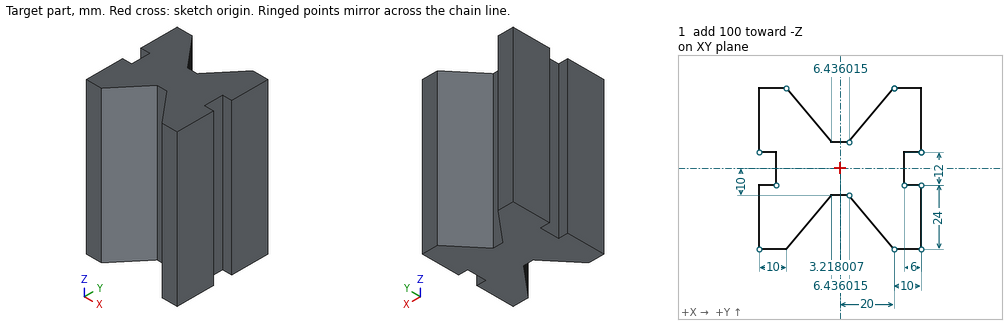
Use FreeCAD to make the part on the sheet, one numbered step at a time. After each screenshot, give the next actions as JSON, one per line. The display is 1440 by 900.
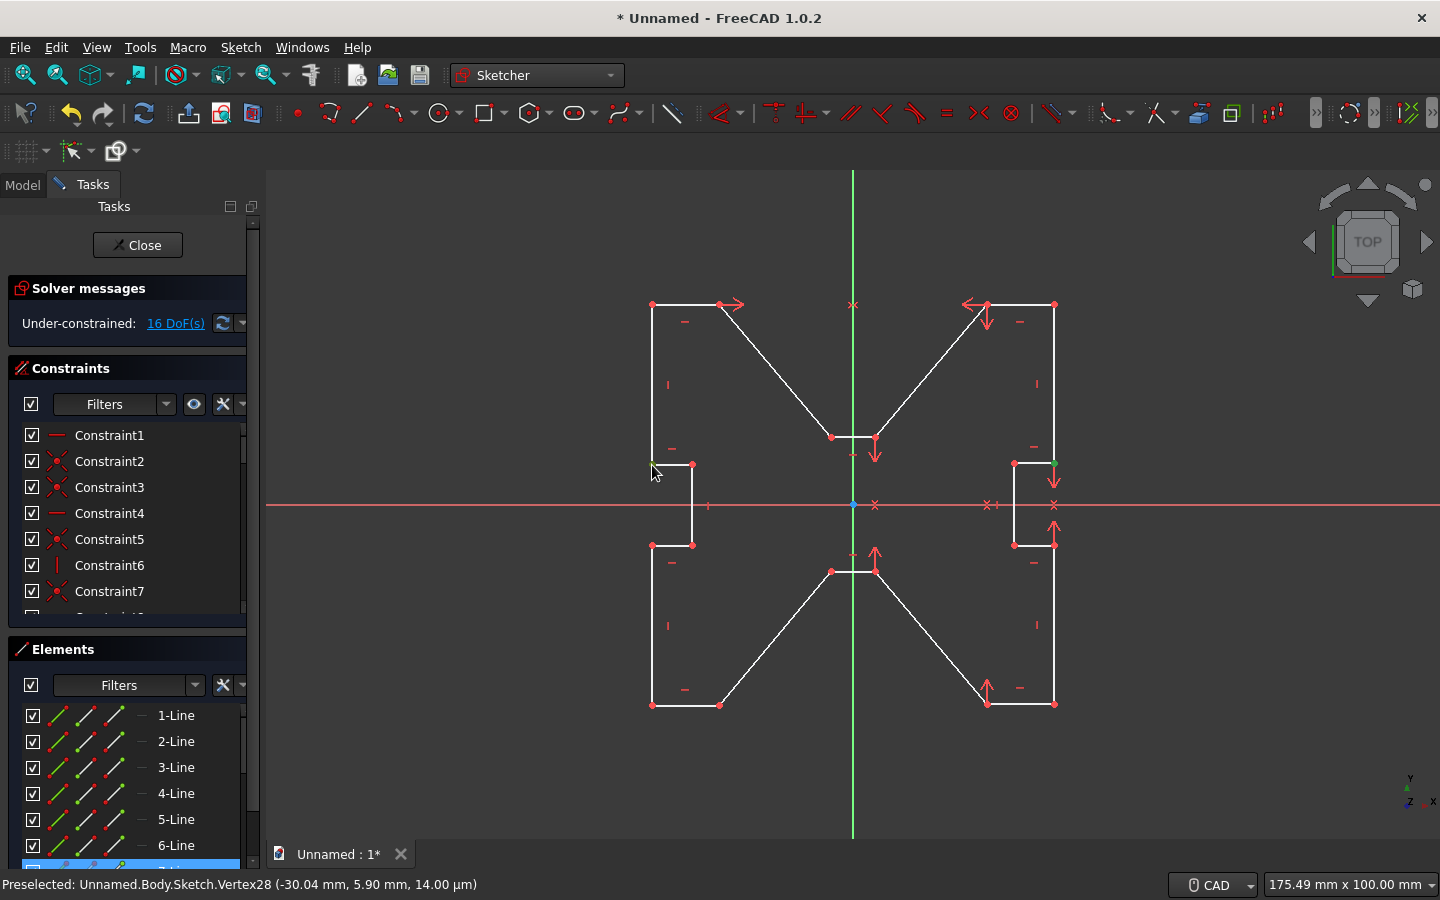
{"action": "left_click", "coordinate": [853, 767]}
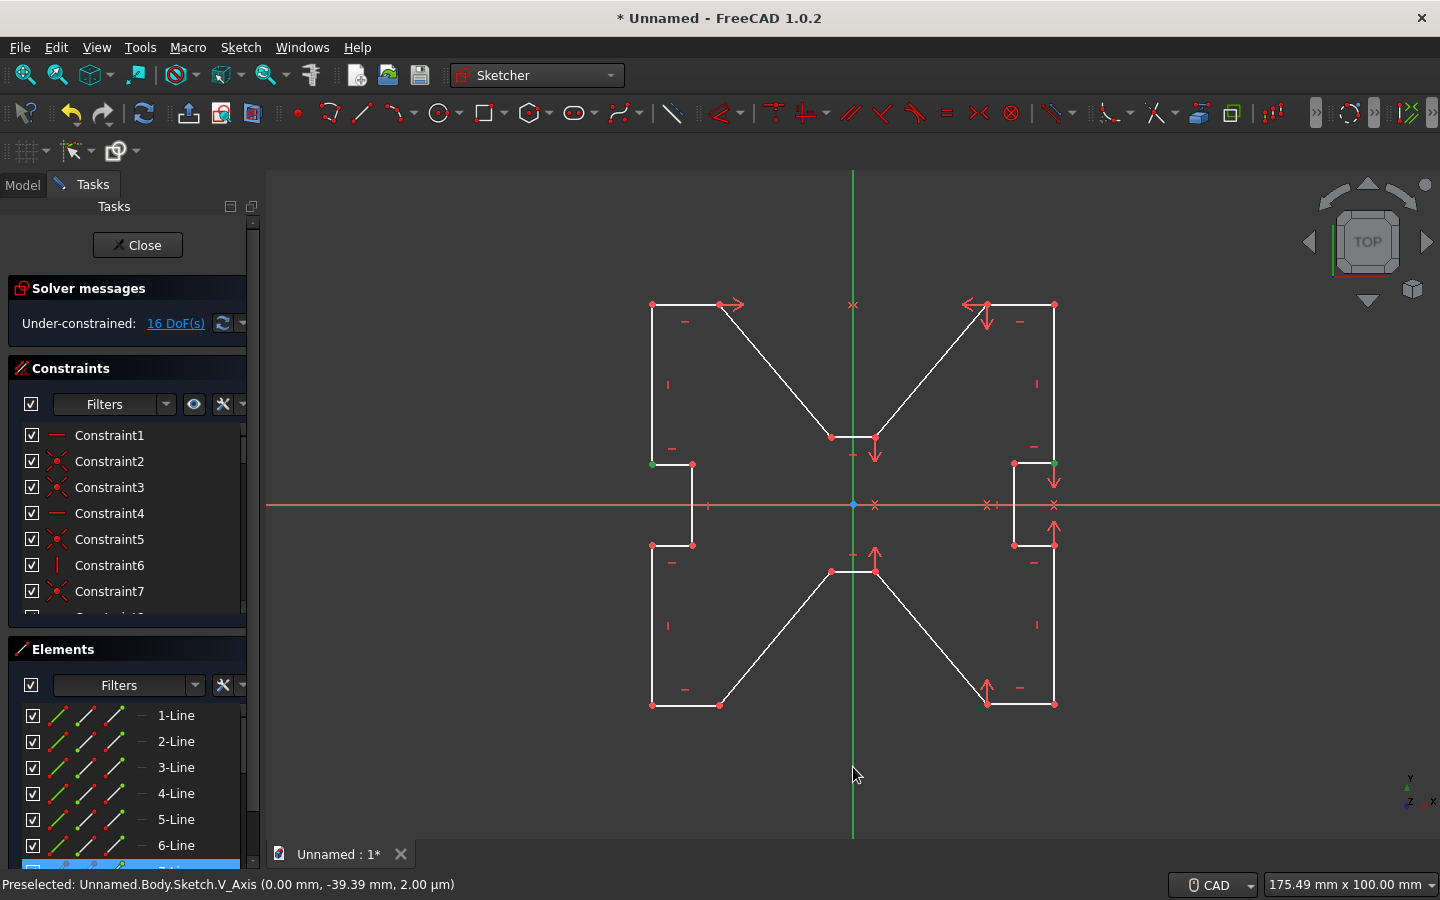
{"action": "left_click", "coordinate": [980, 114]}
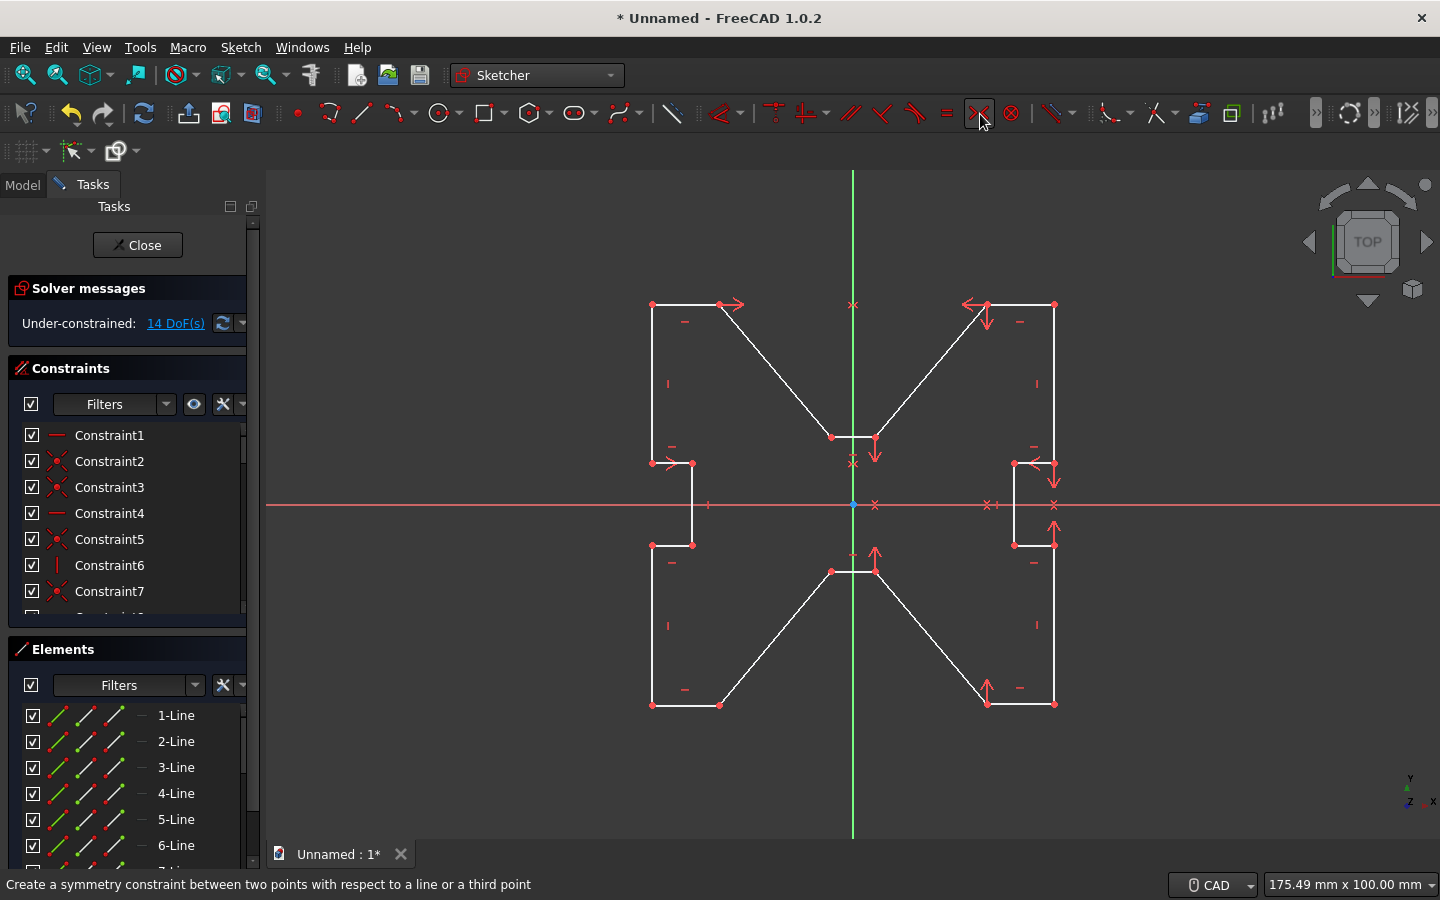
{"action": "left_click", "coordinate": [1014, 546]}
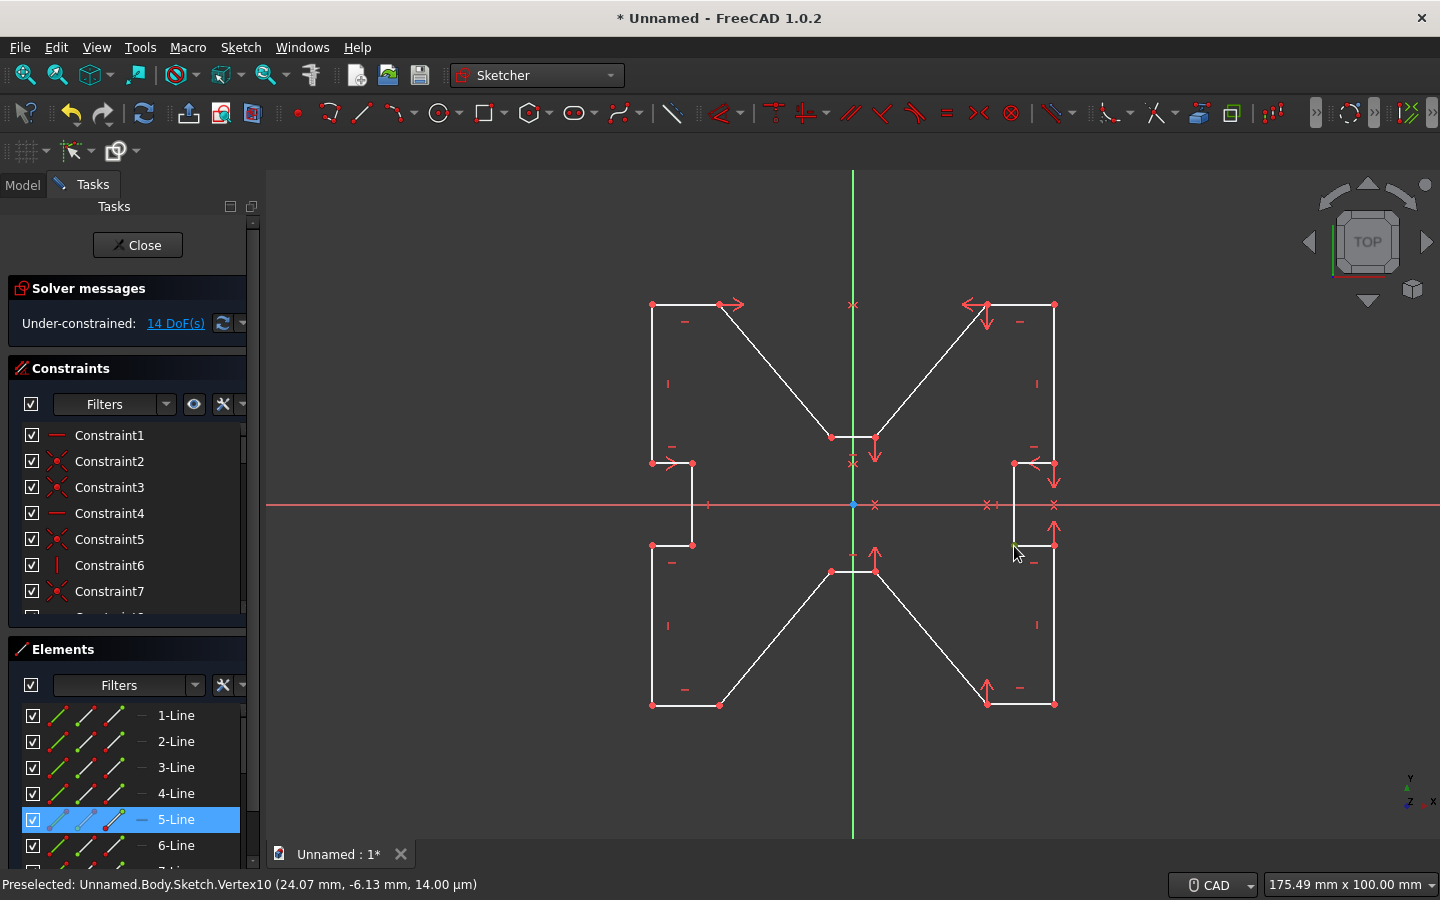
{"action": "left_click", "coordinate": [692, 546]}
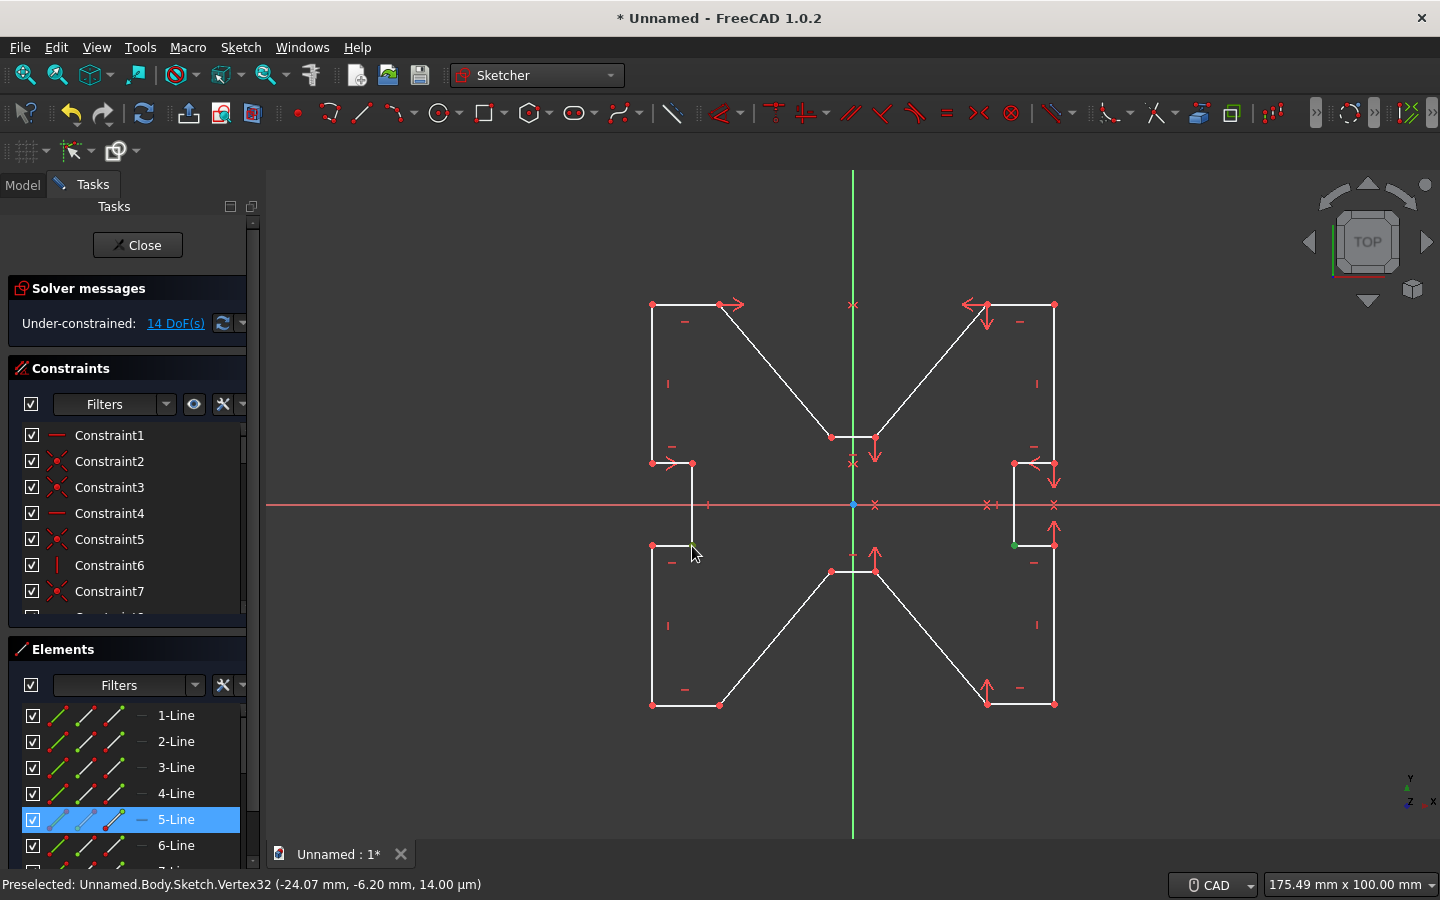
{"action": "left_click", "coordinate": [853, 767]}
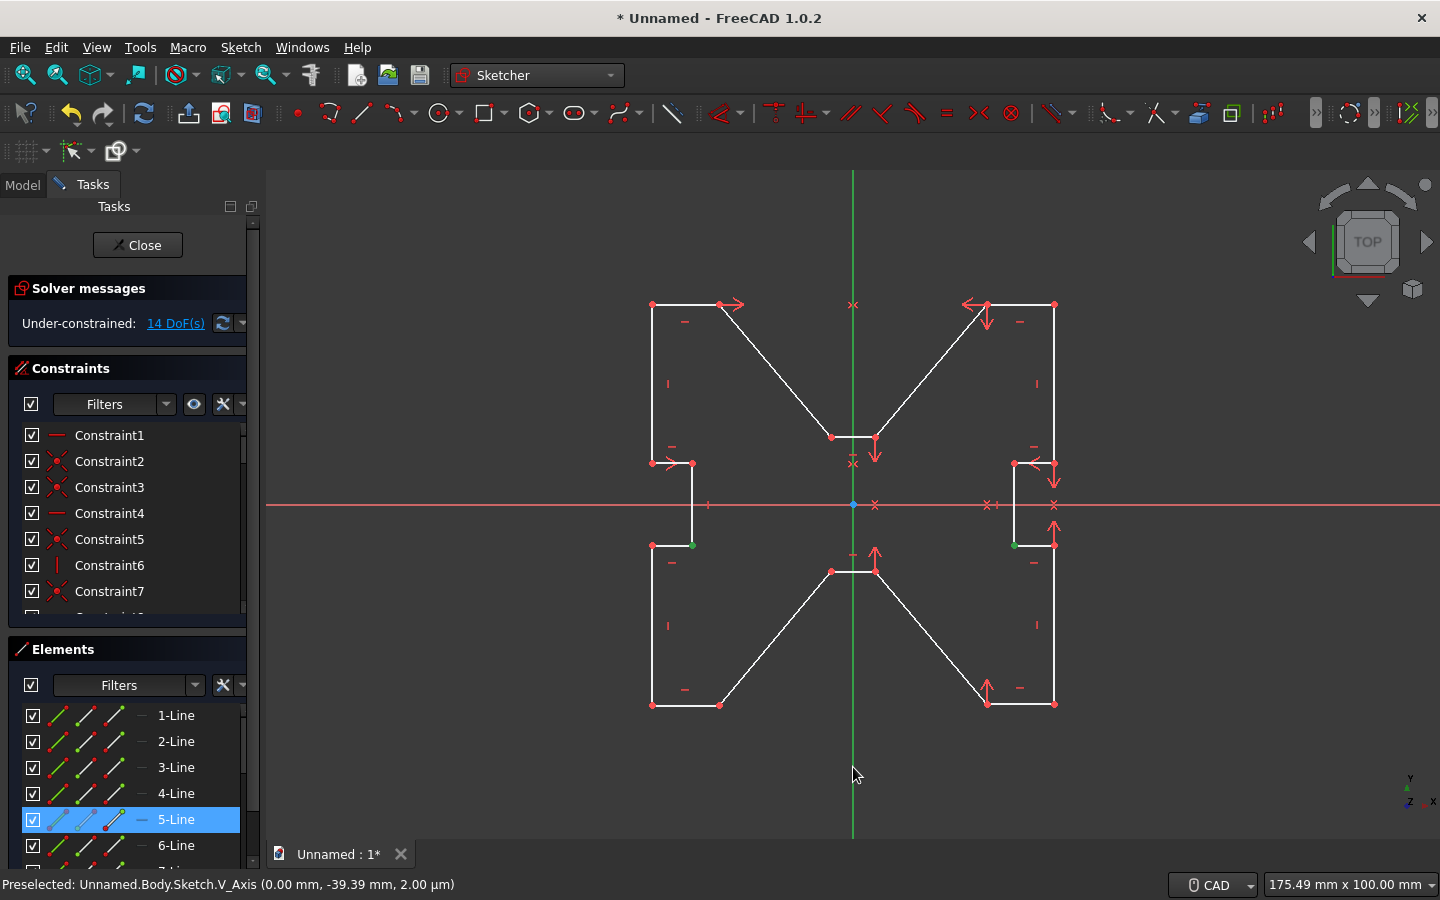
{"action": "key", "text": "s"}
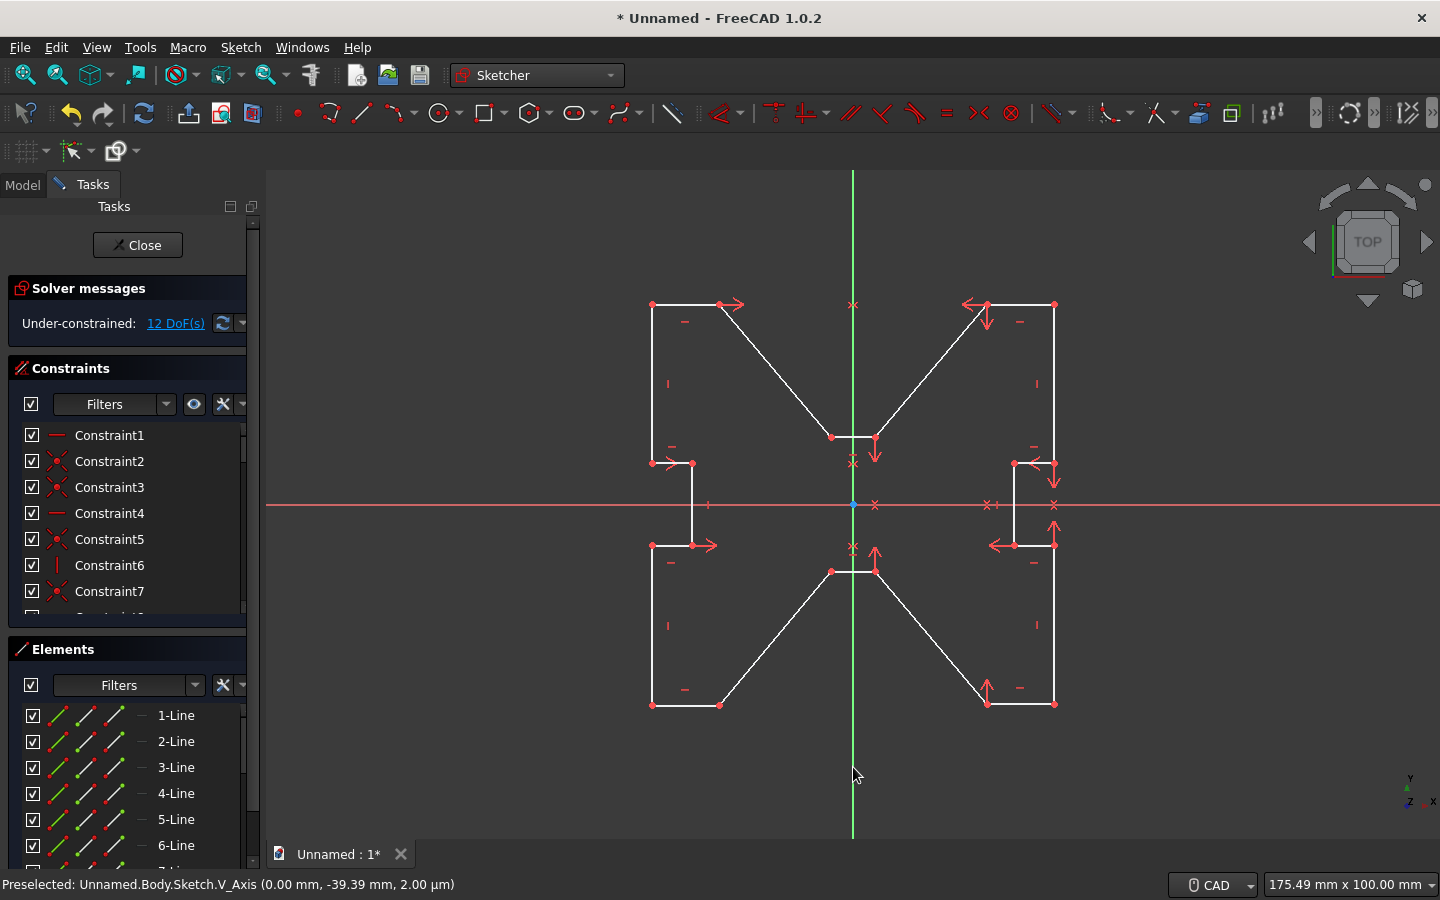
{"action": "left_click", "coordinate": [1054, 704]}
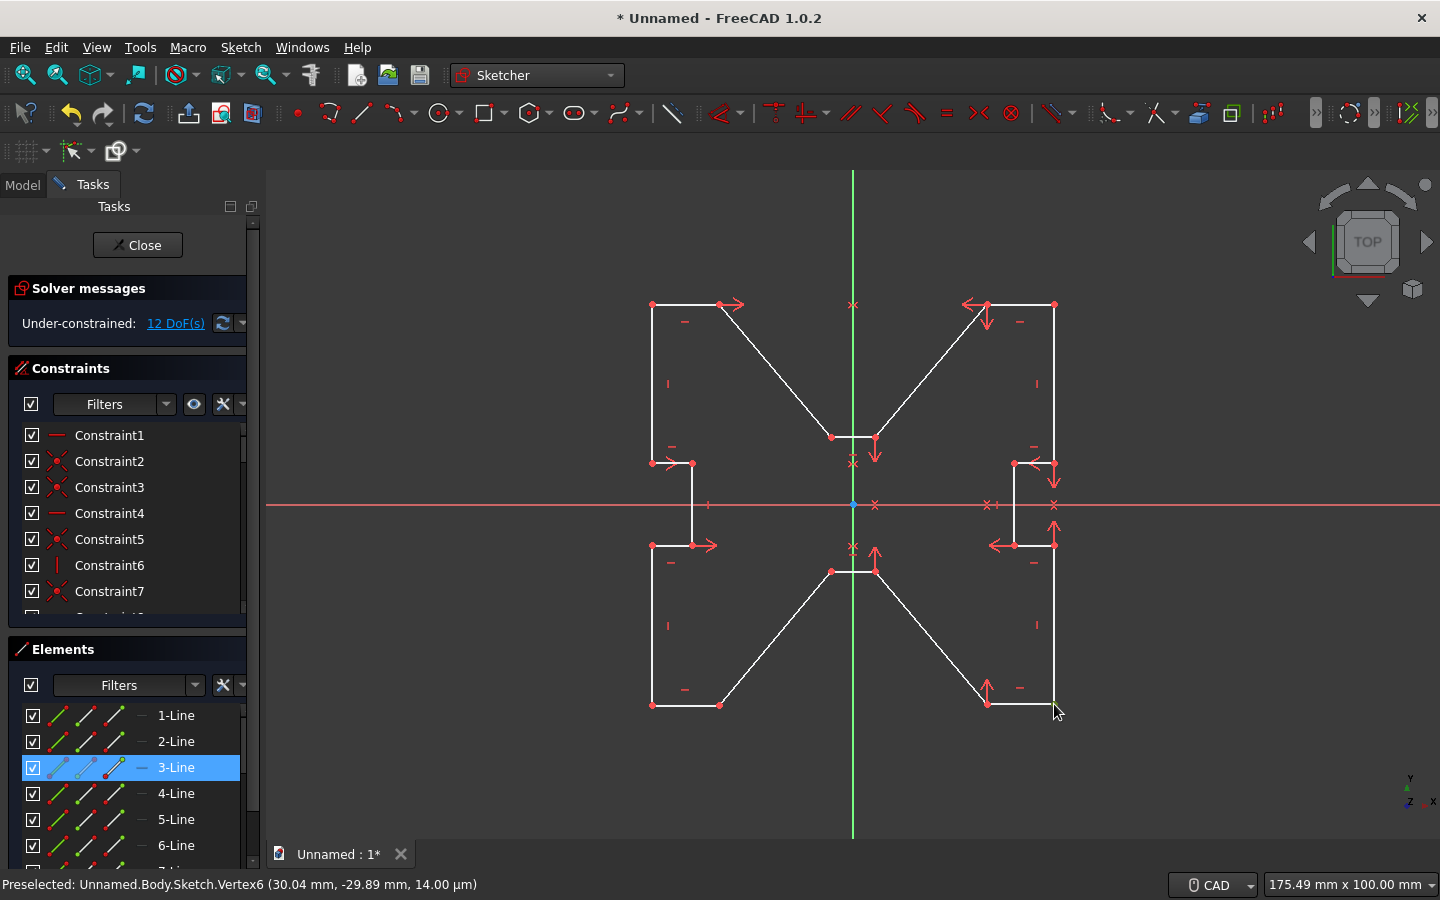
{"action": "left_click", "coordinate": [652, 706]}